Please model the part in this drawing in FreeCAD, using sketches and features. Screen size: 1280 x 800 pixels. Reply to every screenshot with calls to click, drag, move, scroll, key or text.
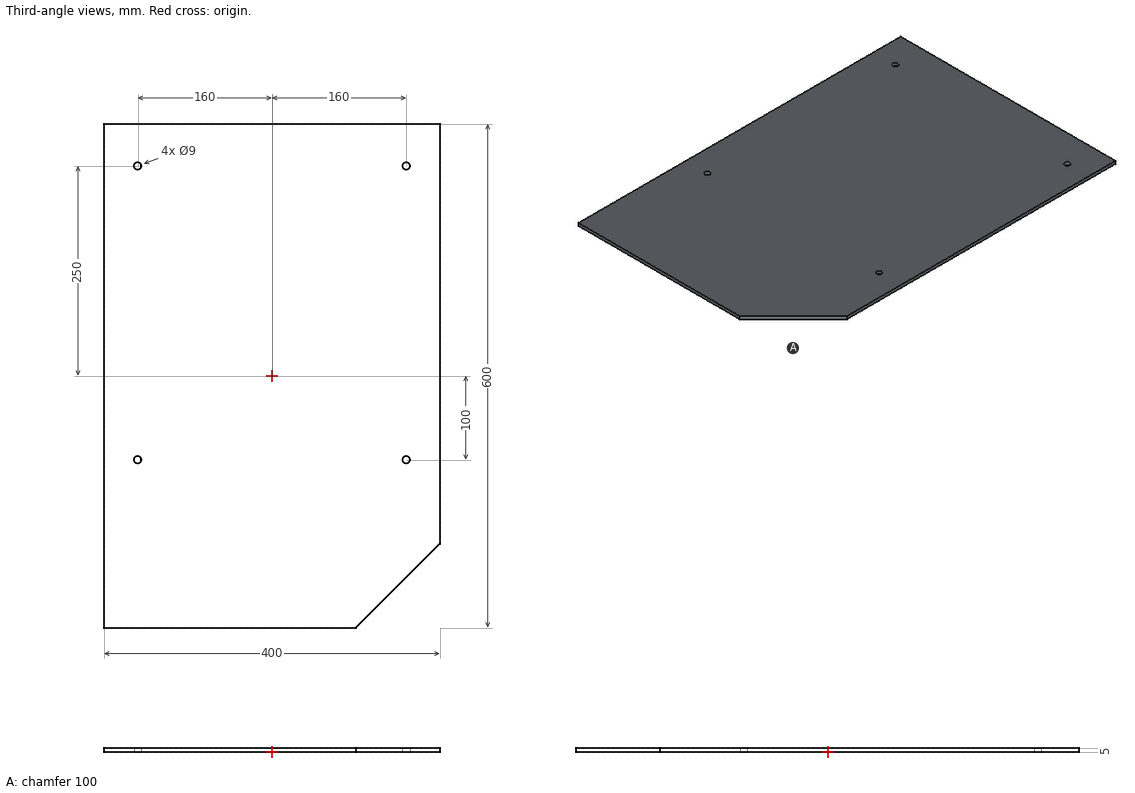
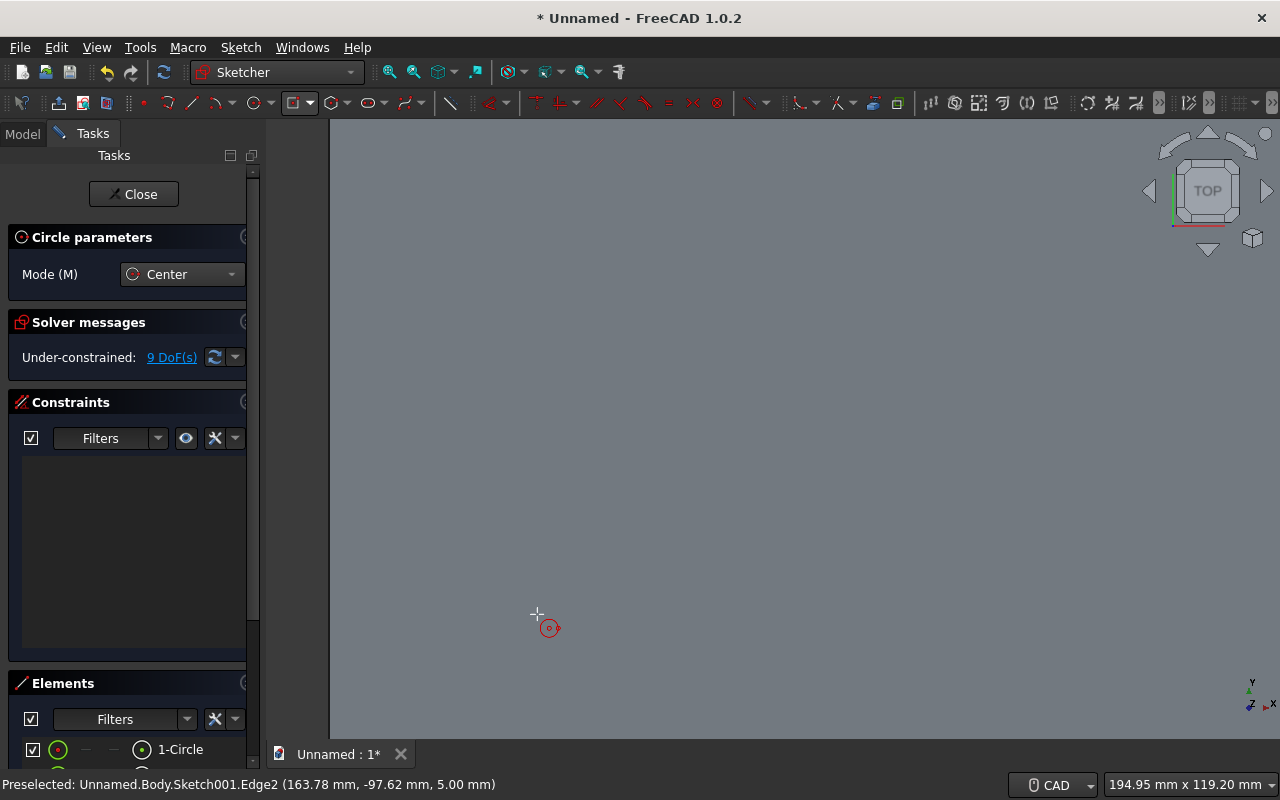
scroll(536, 614, down, 8)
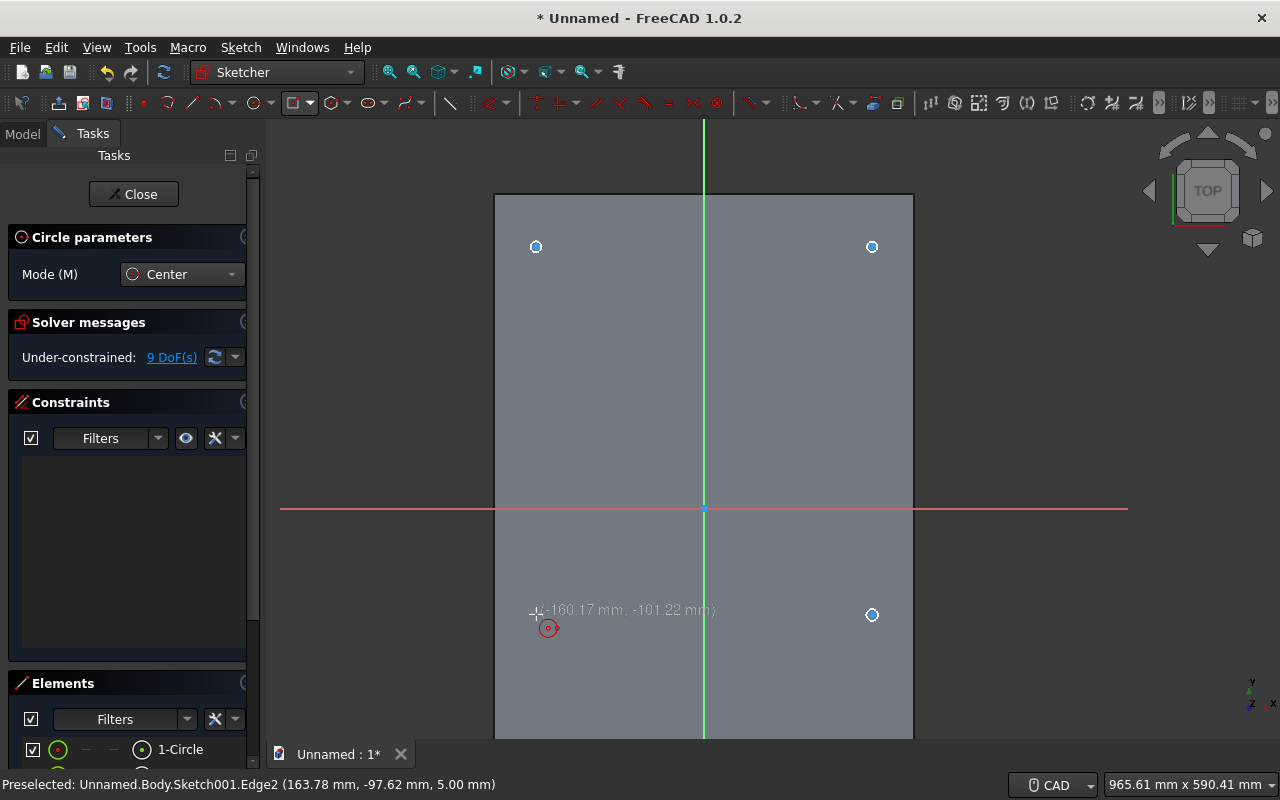
click(536, 614)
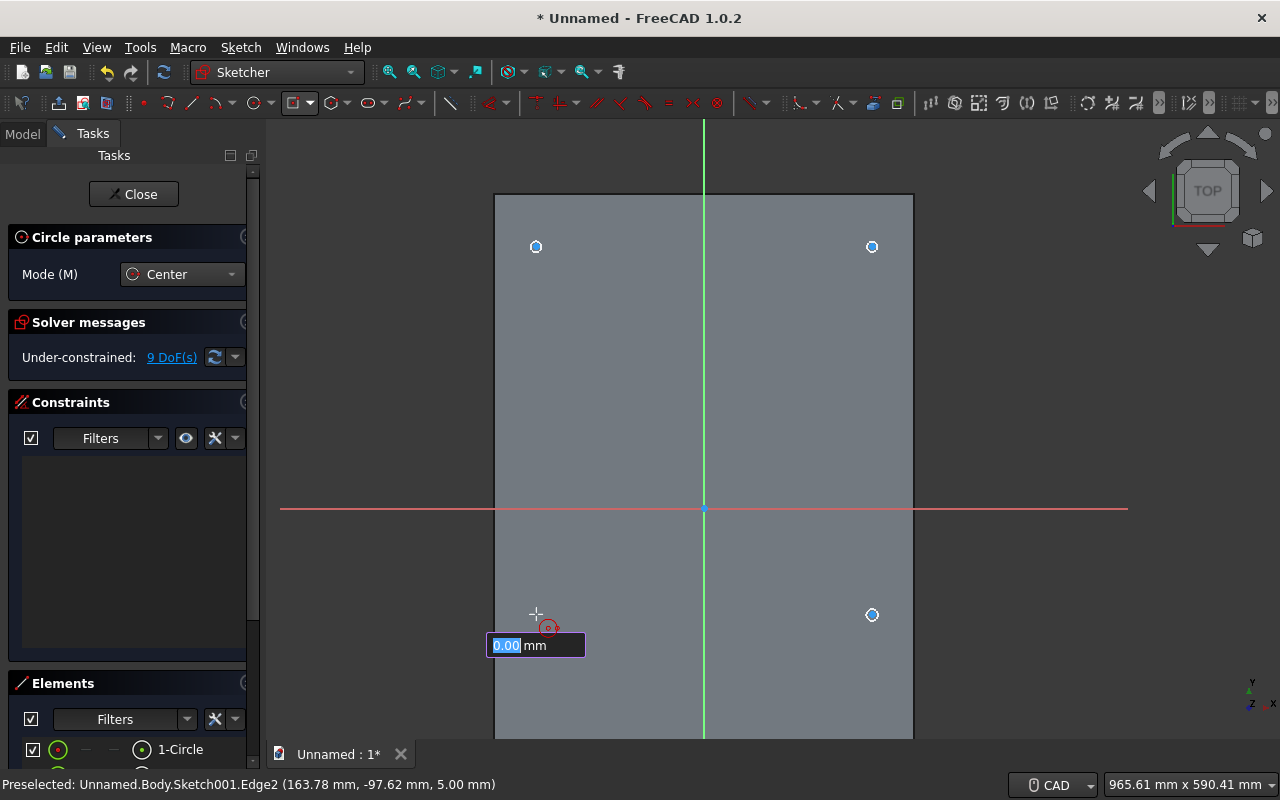
scroll(540, 610, up, 7)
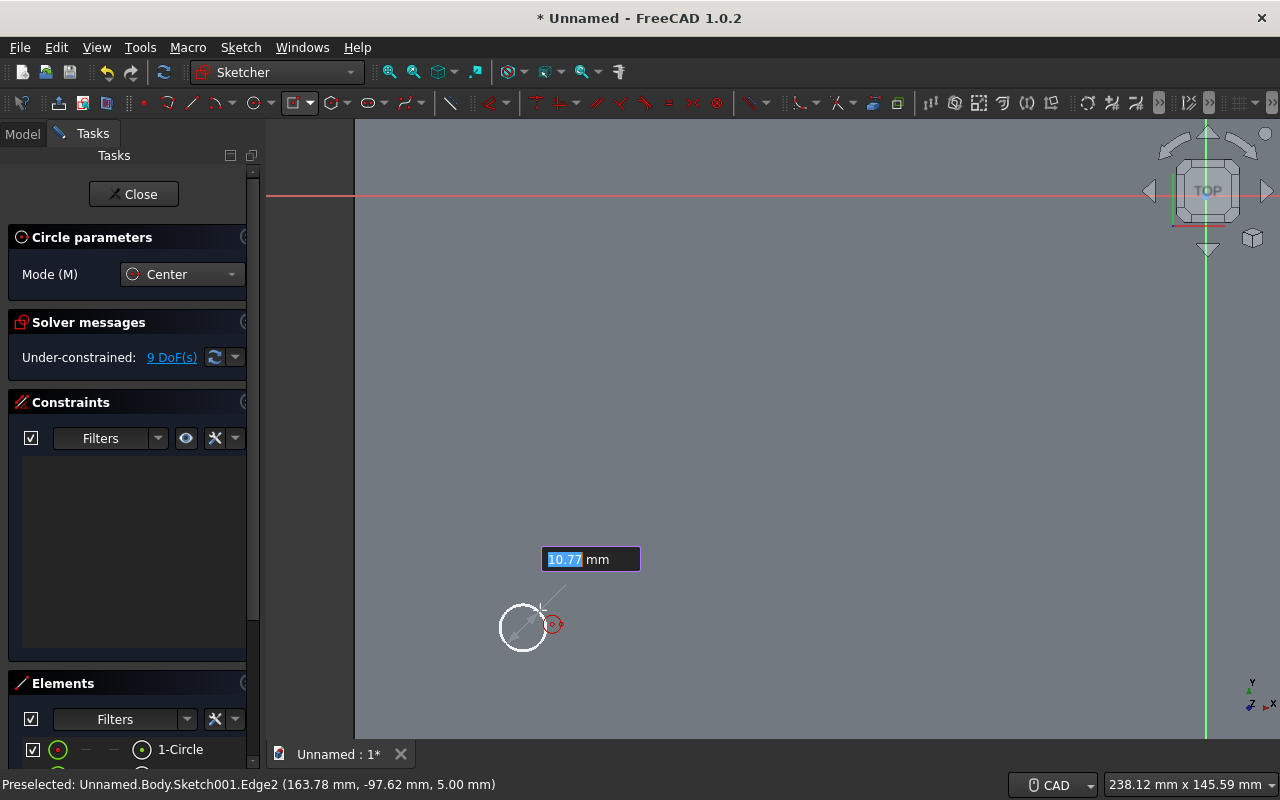
click(538, 608)
key(Escape)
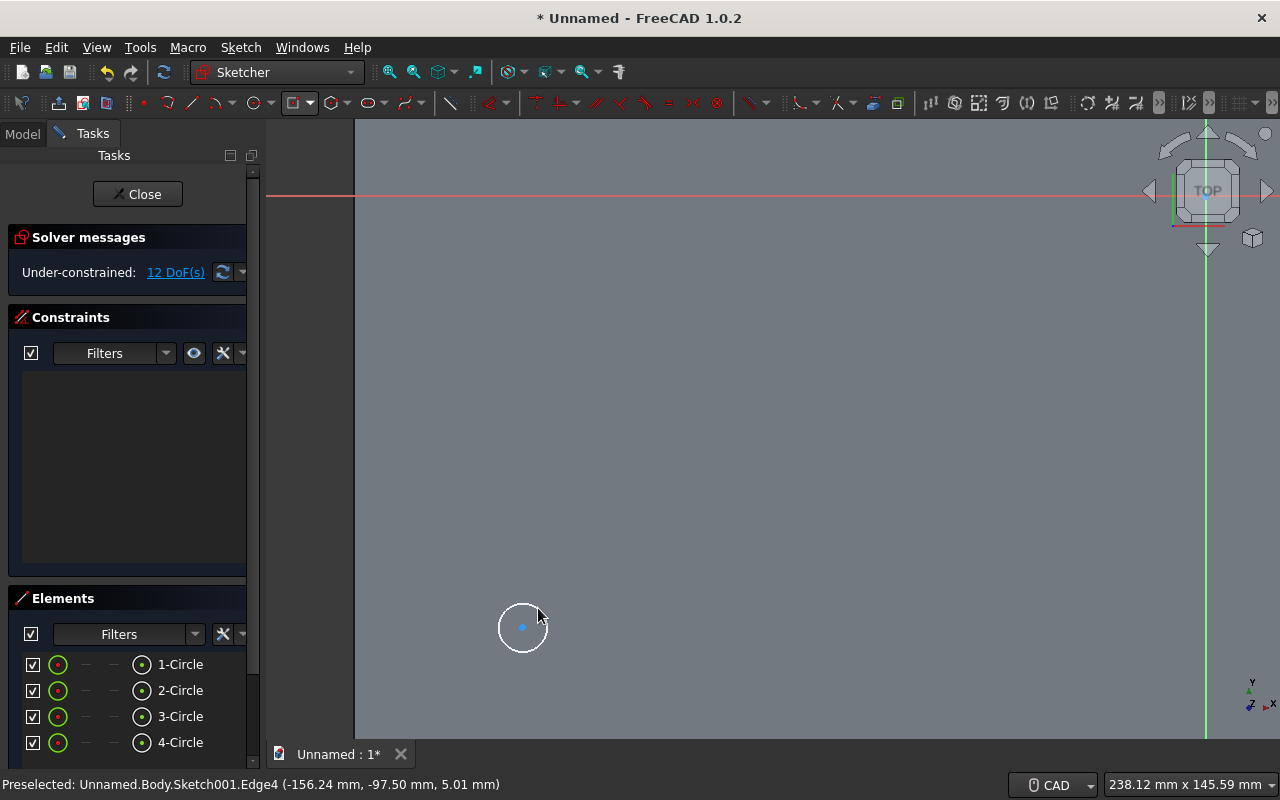
scroll(540, 610, down, 7)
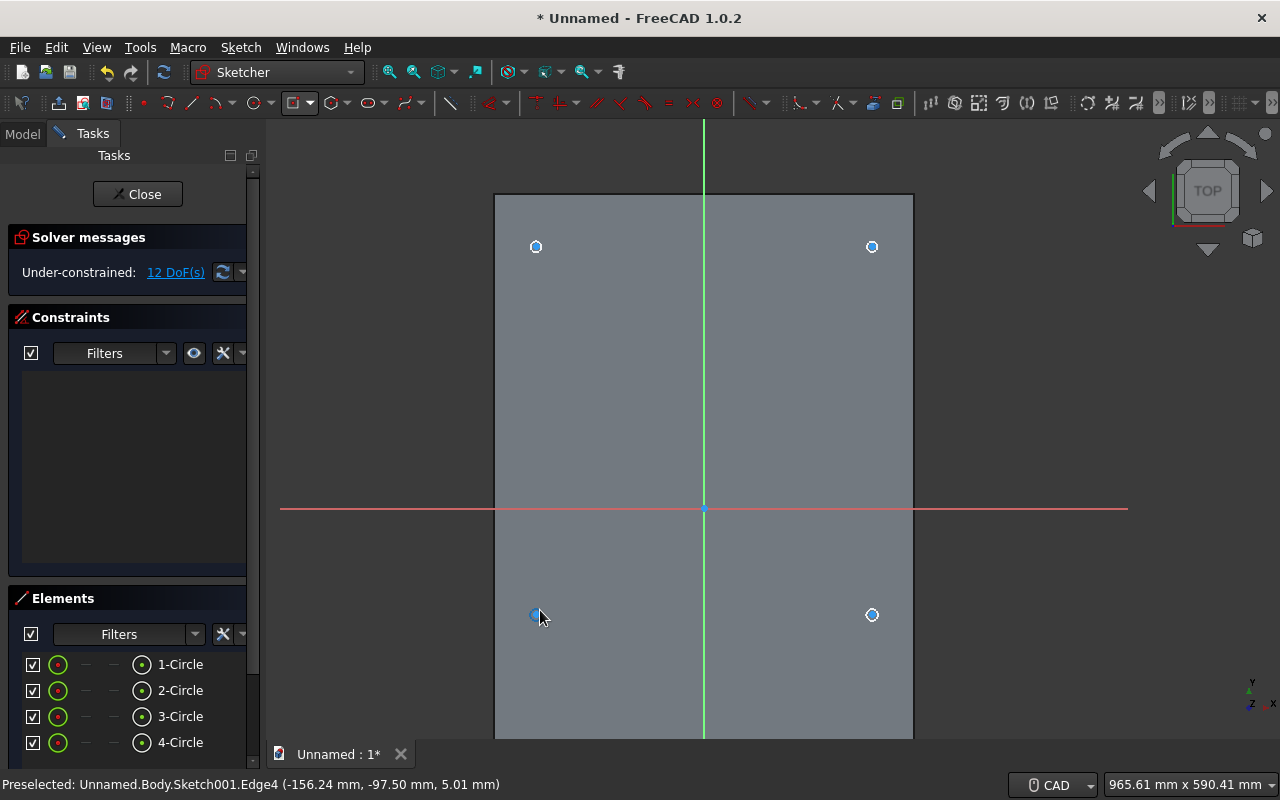
scroll(540, 243, up, 5)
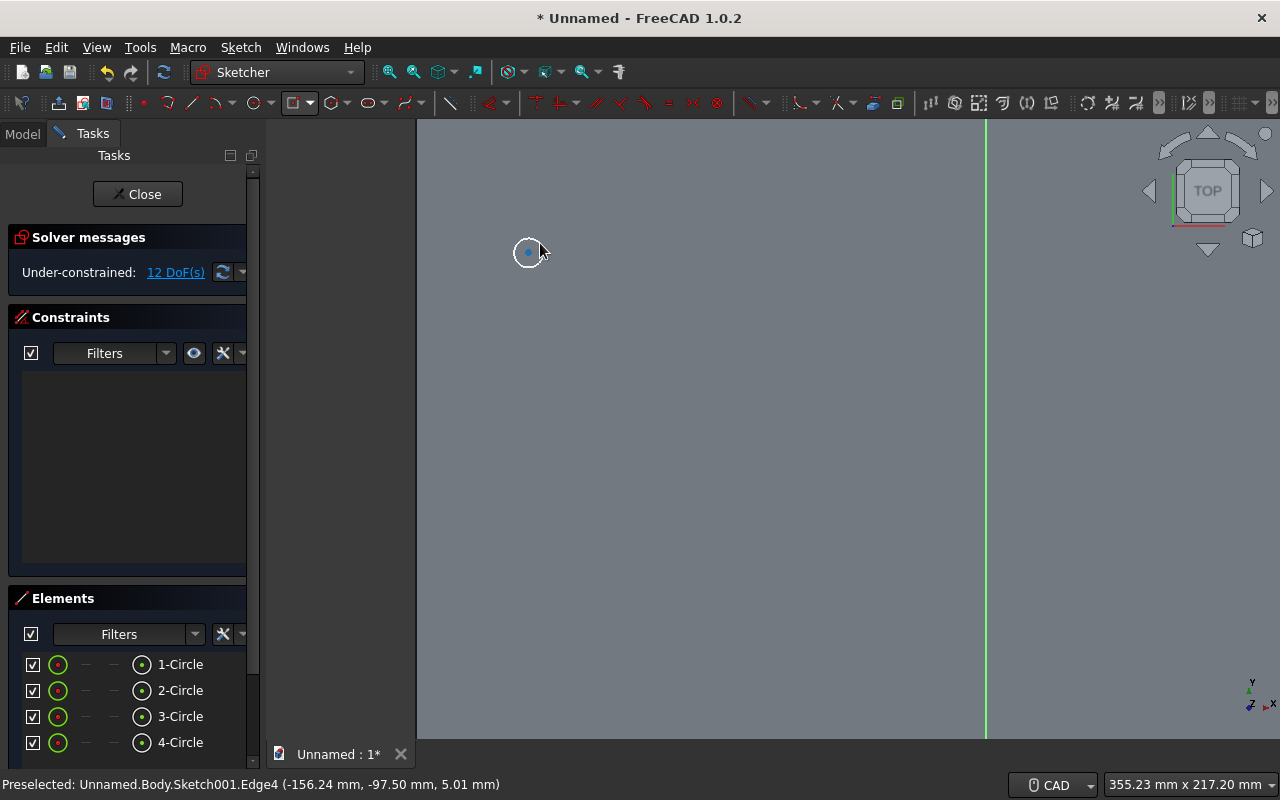
click(539, 243)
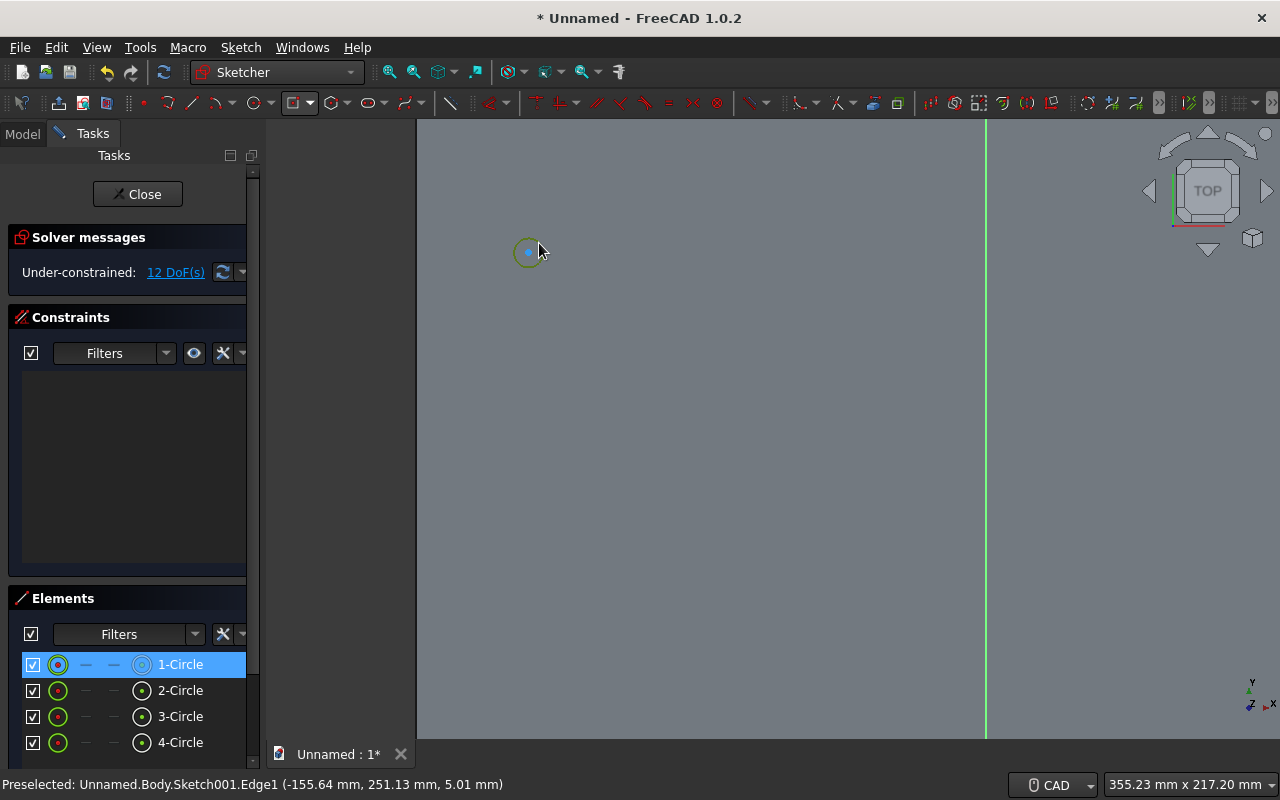
scroll(540, 242, down, 5)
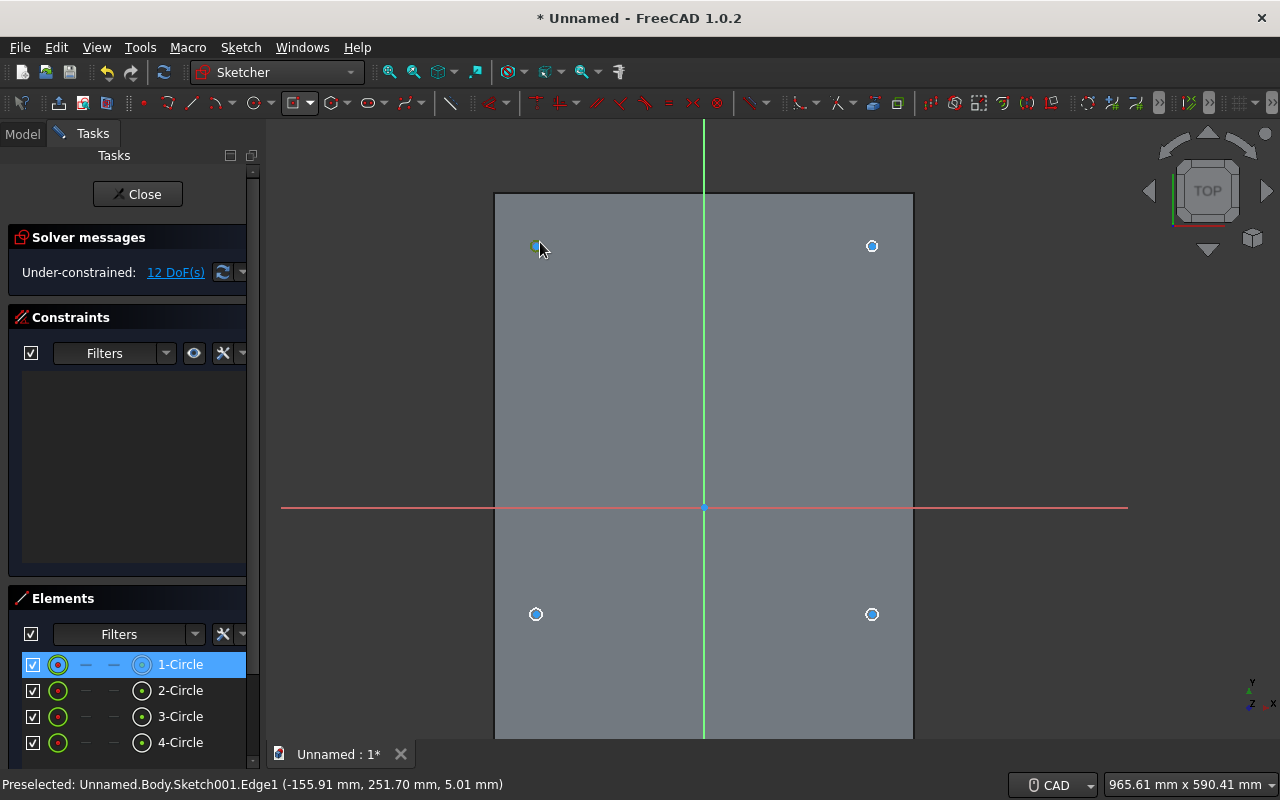
scroll(876, 242, up, 5)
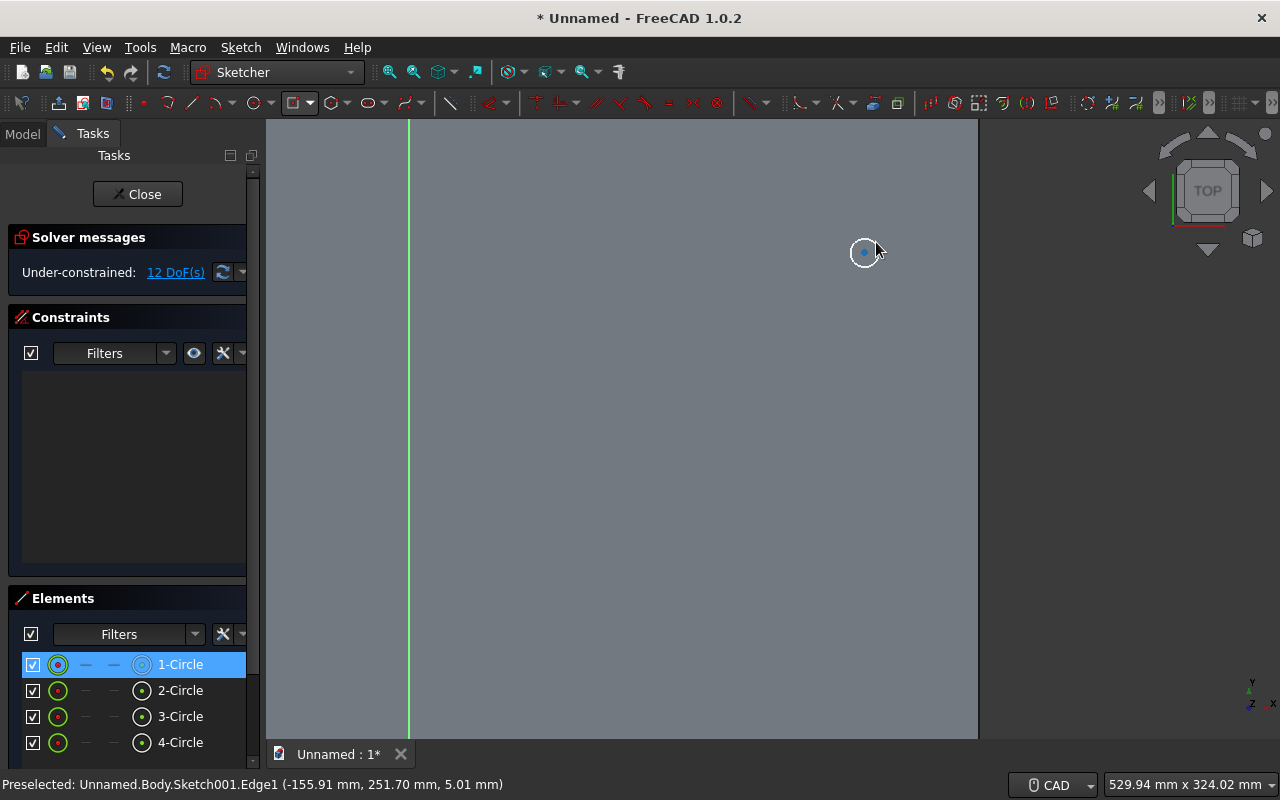
click(875, 243)